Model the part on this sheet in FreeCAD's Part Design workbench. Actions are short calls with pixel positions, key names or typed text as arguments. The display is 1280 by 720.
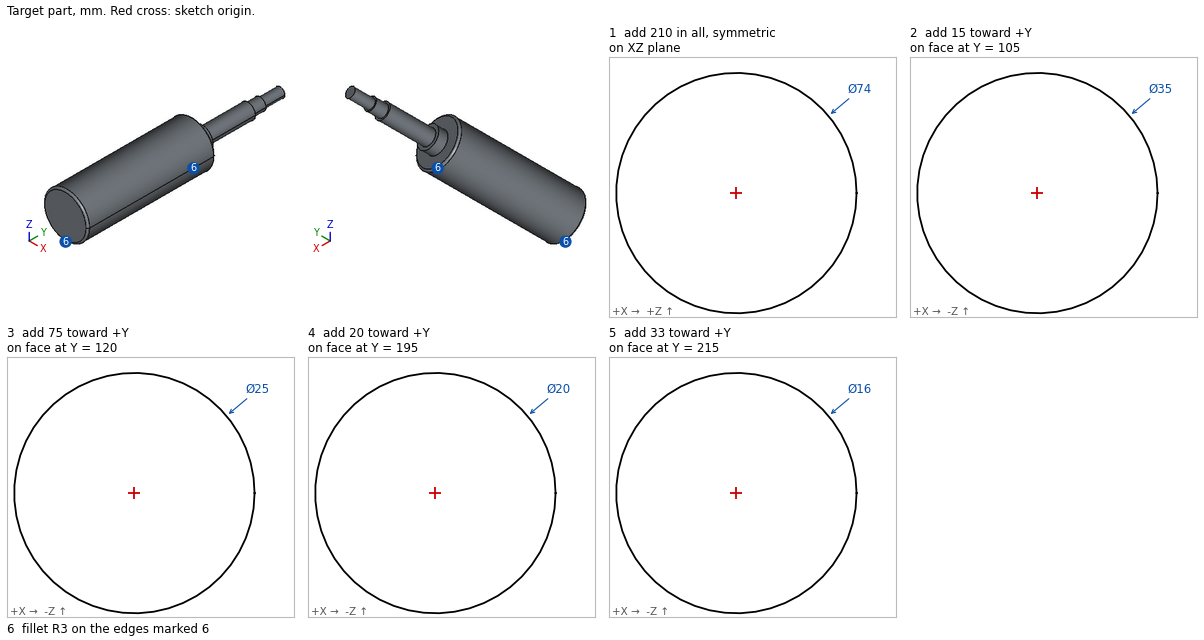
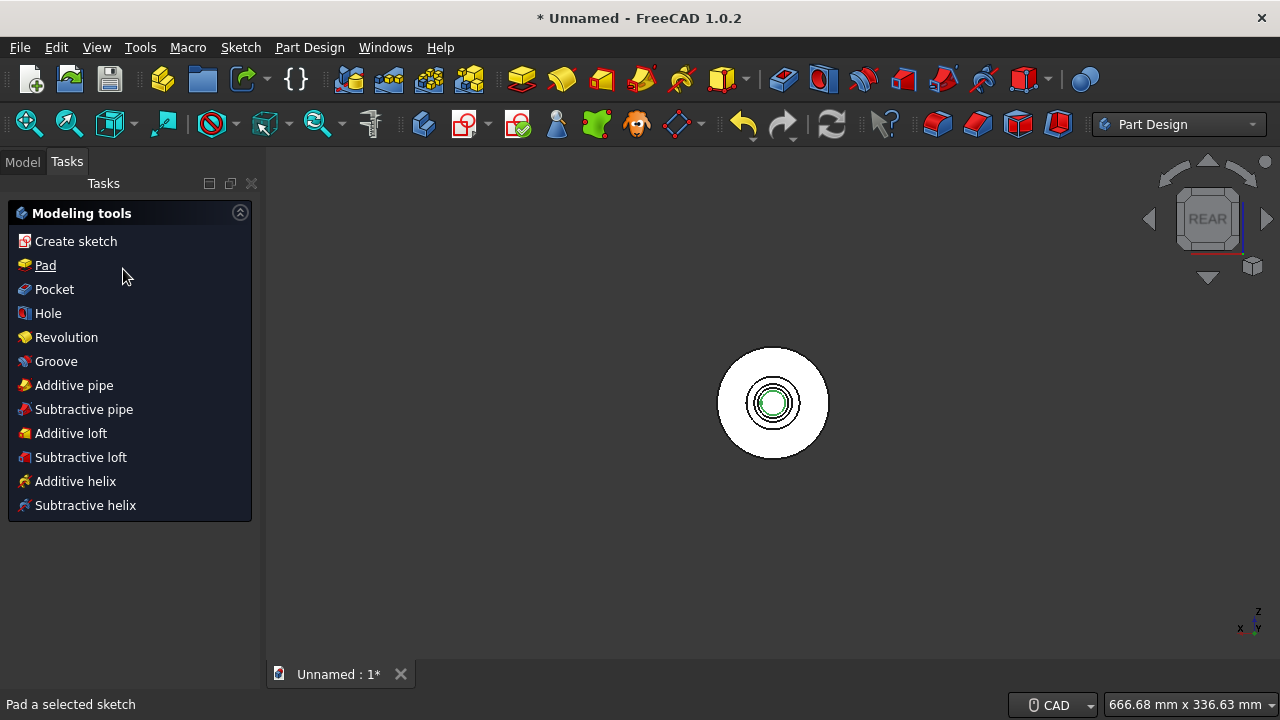
click(522, 80)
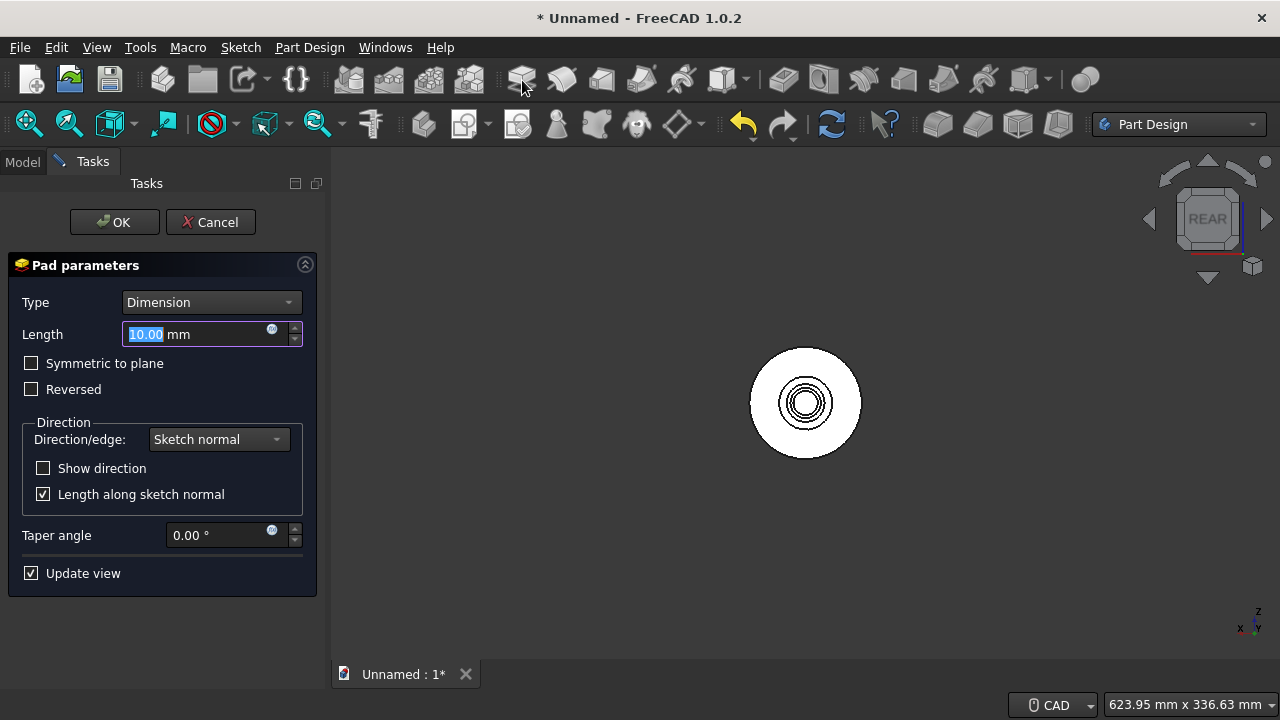
text(33)
key(Tab)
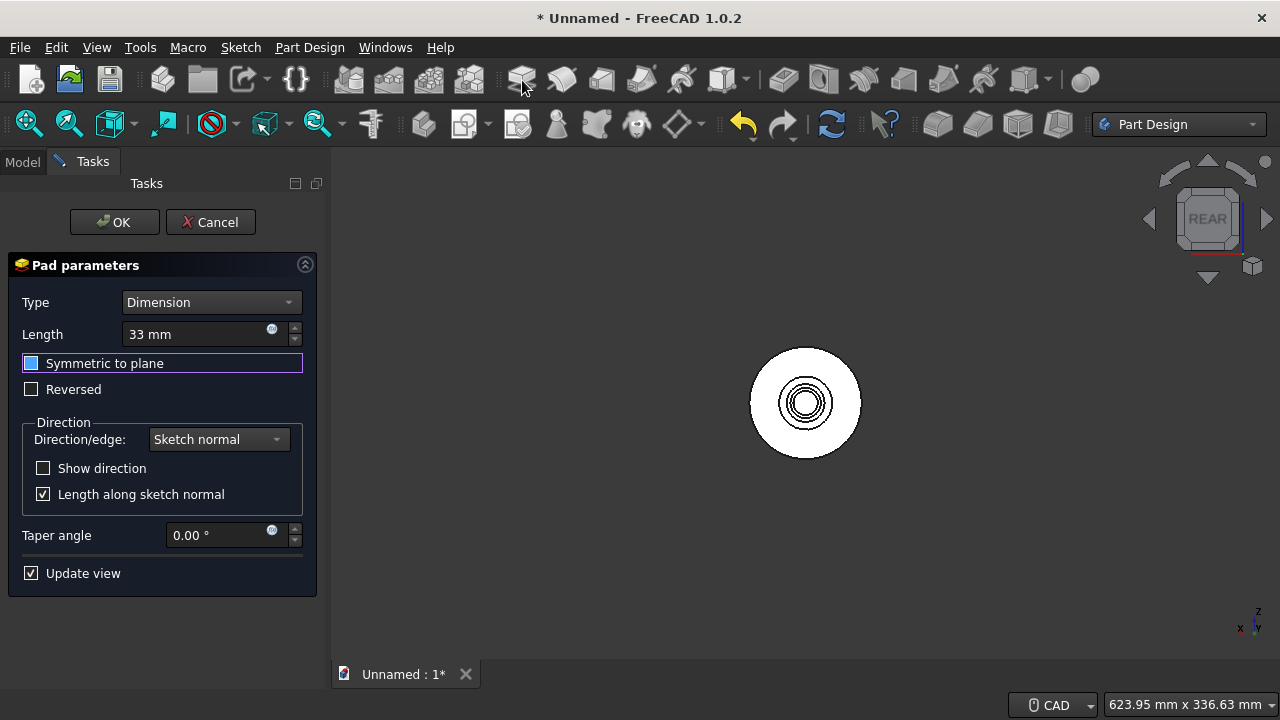
click(115, 222)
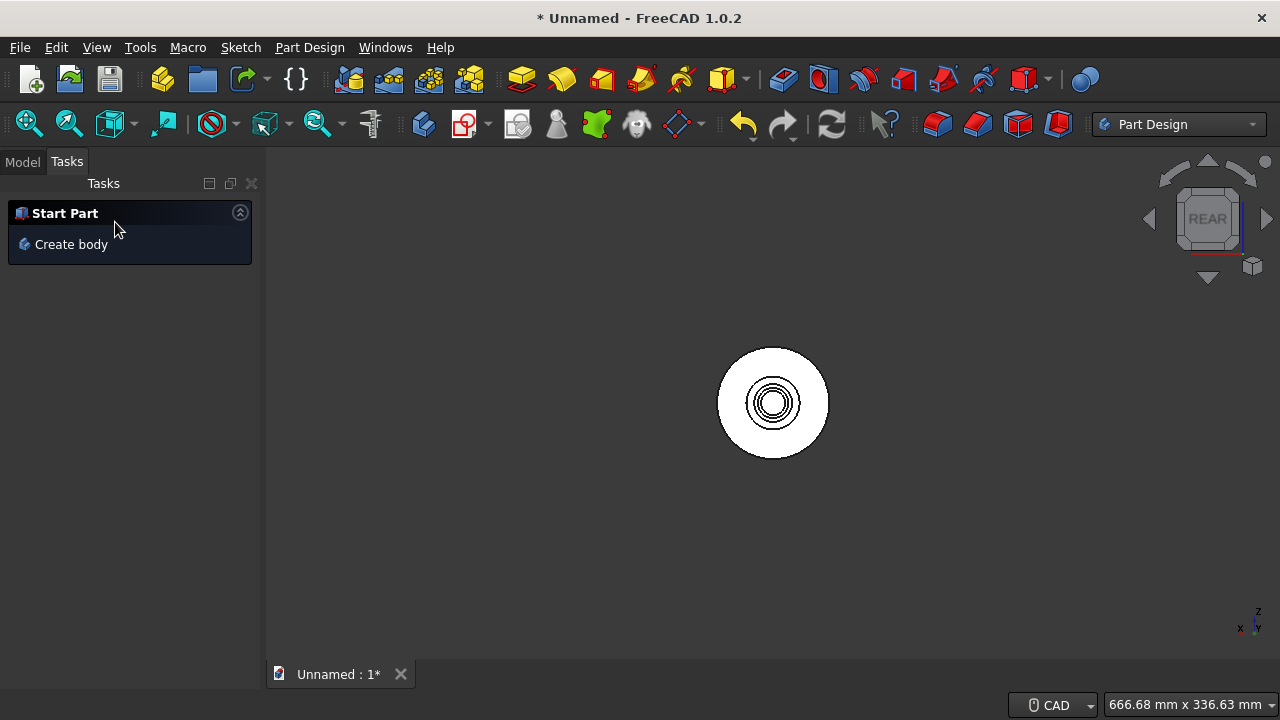
click(30, 124)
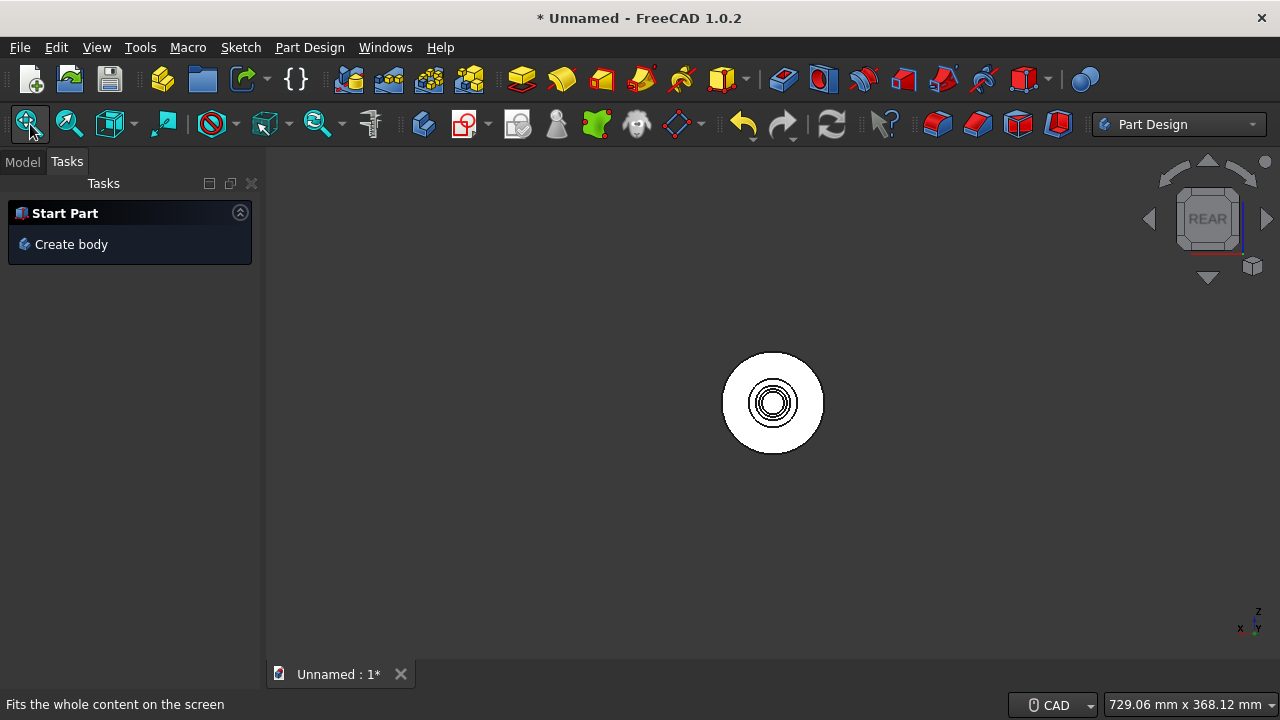
click(824, 402)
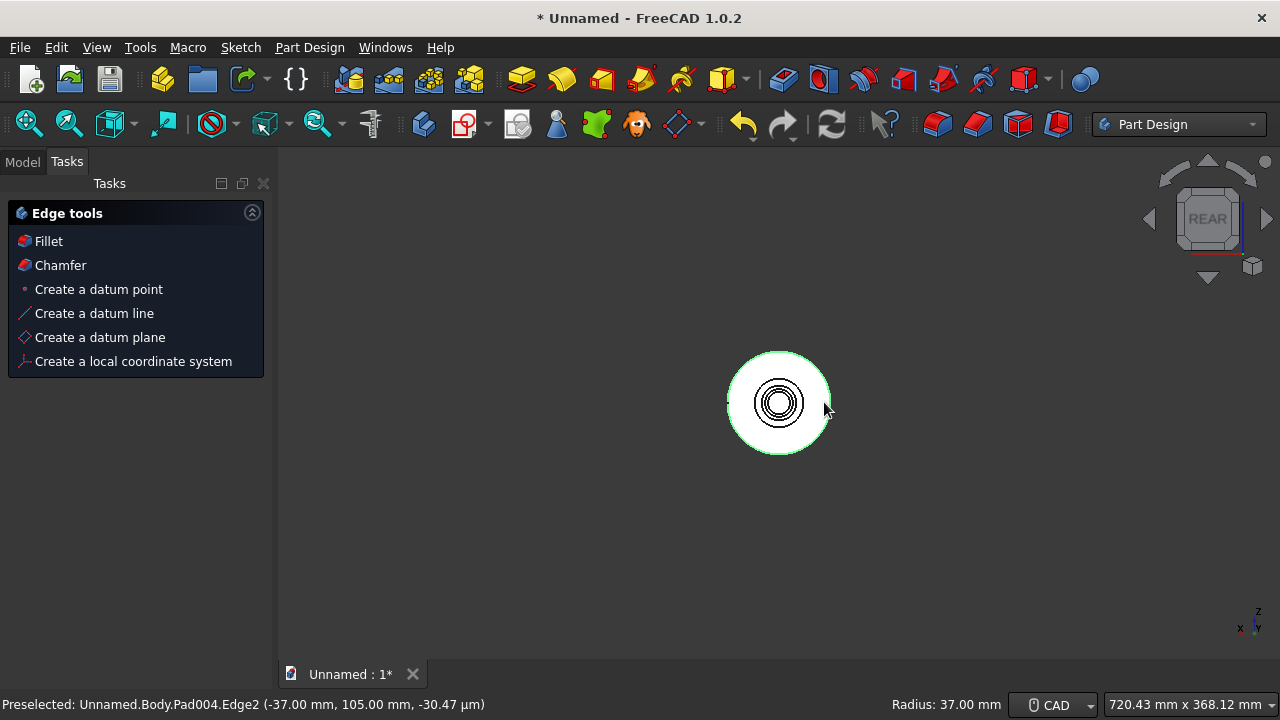
key(0)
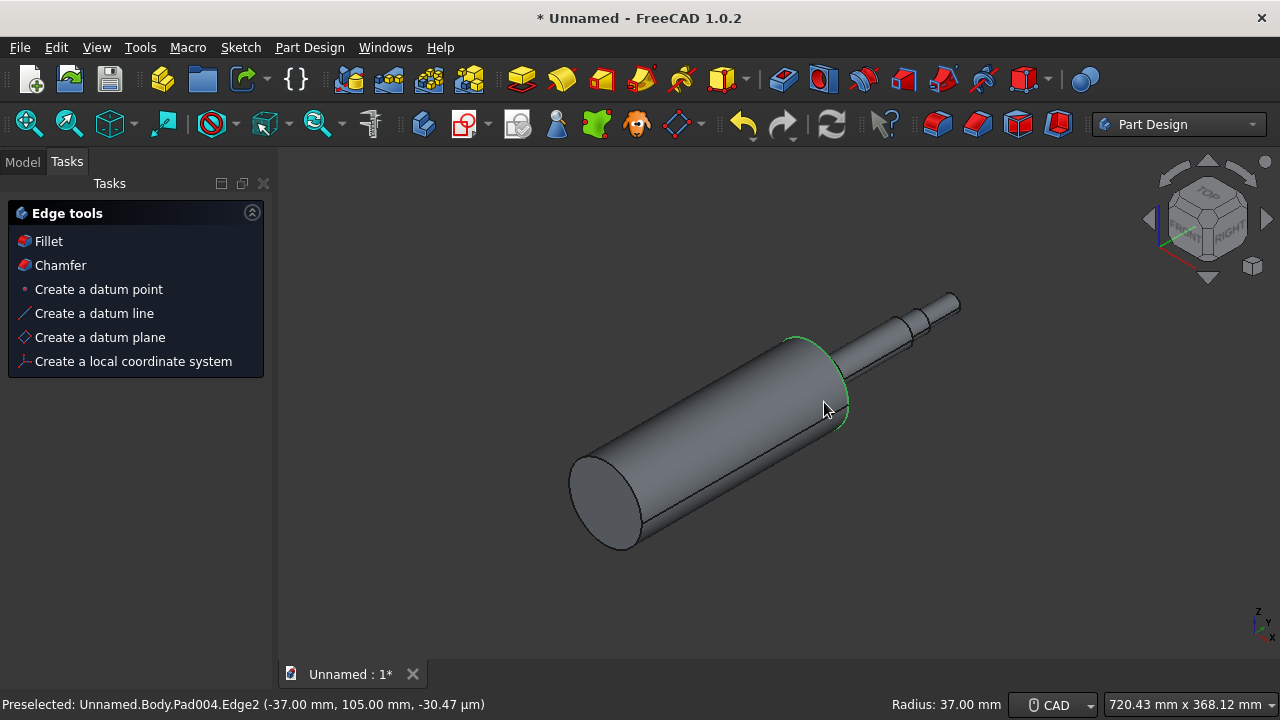
click(594, 456, ctrl)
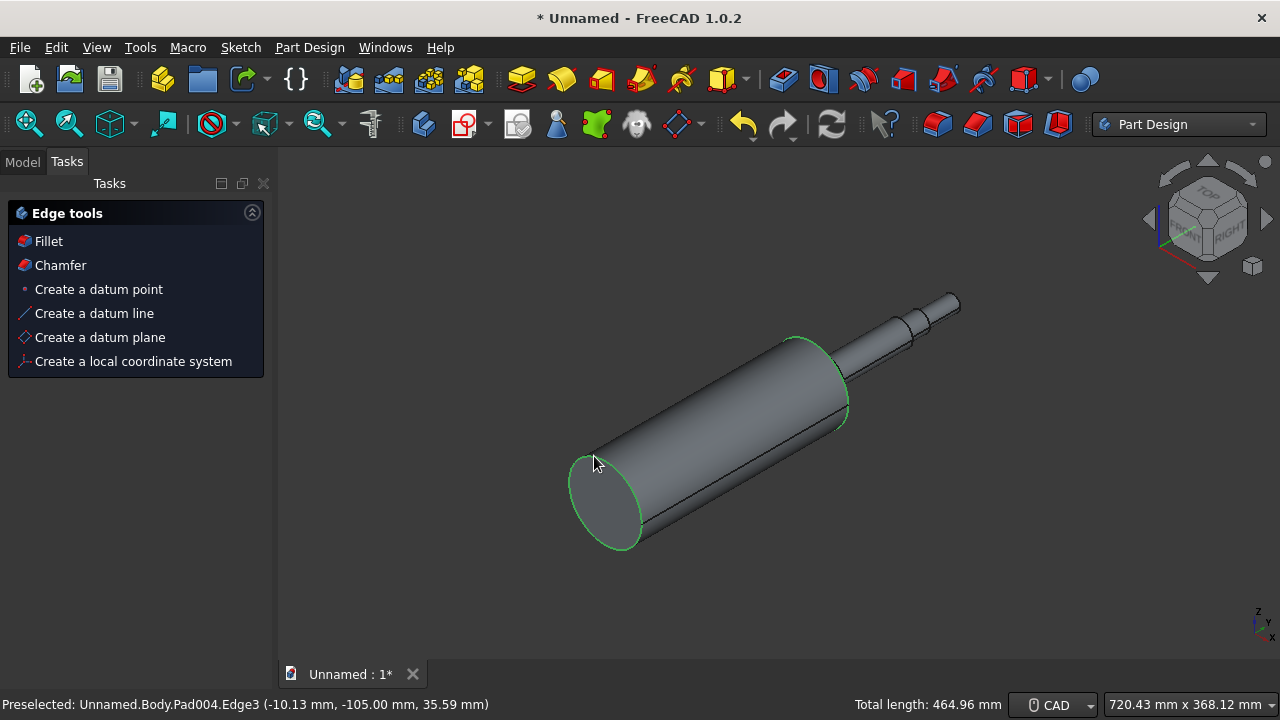
click(938, 124)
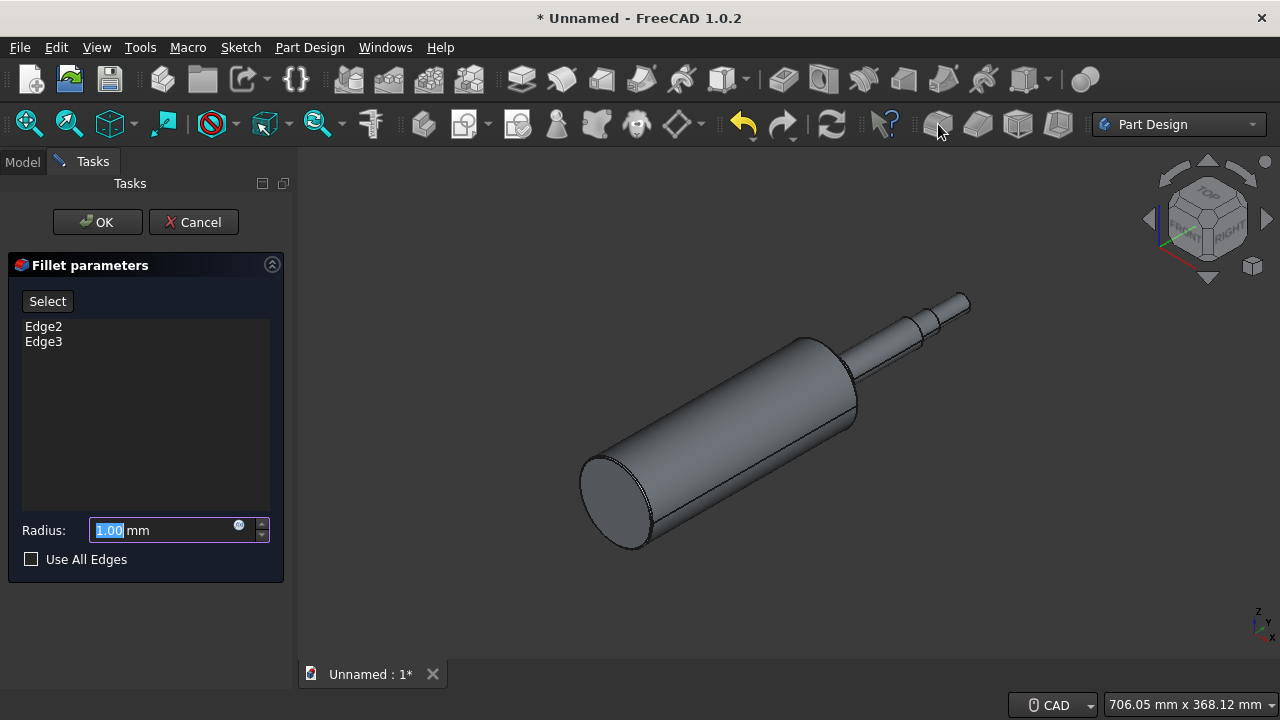
text(3)
key(Tab)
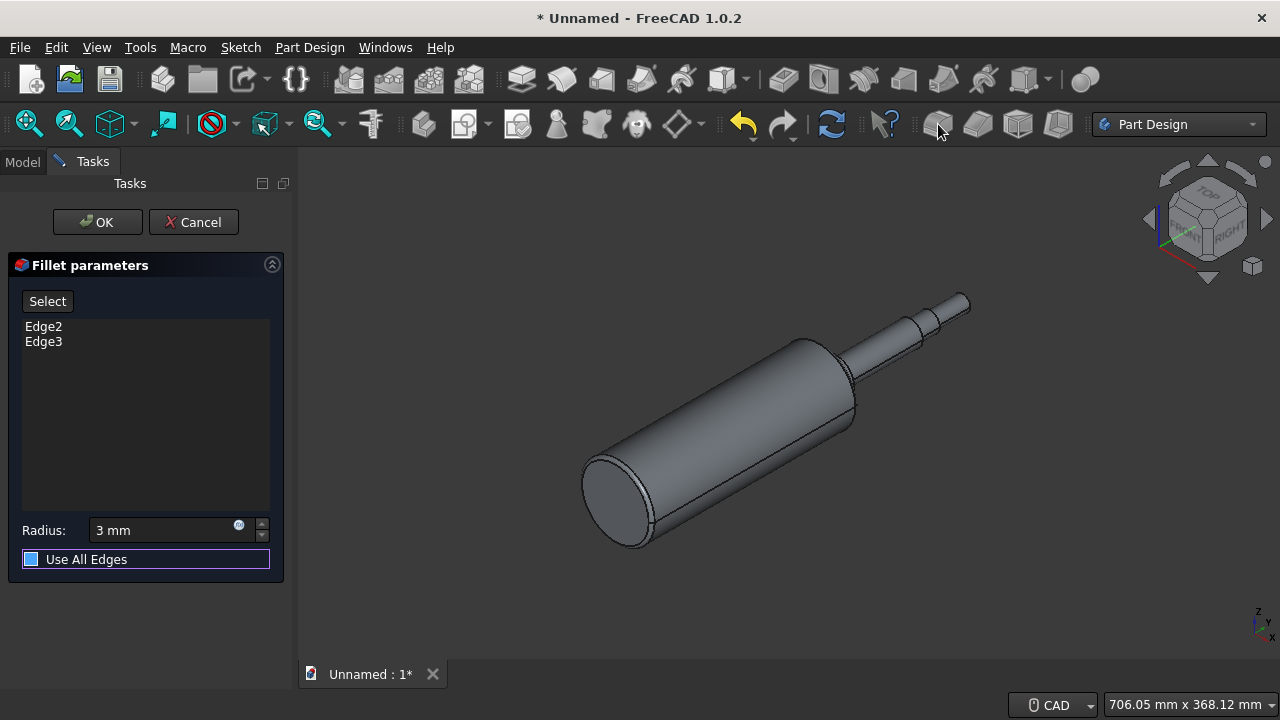
click(98, 222)